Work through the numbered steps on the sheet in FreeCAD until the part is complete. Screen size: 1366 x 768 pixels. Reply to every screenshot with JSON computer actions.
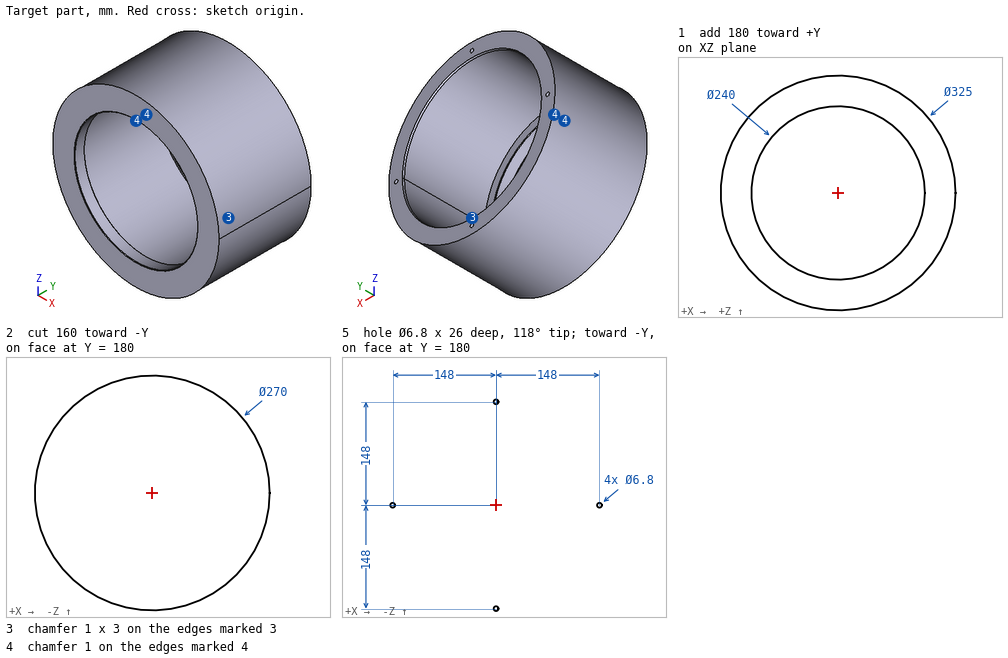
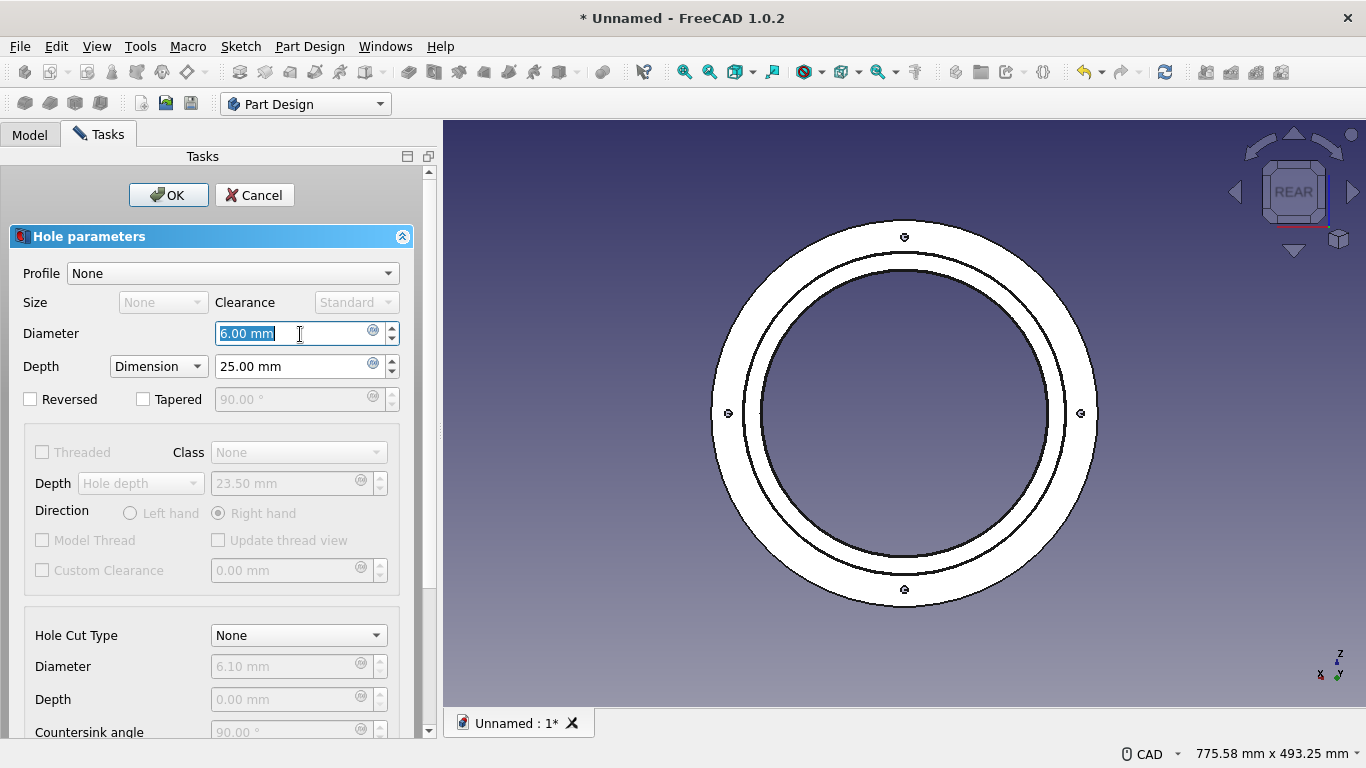
{"action": "type", "text": "6.8"}
{"action": "key", "text": "Tab"}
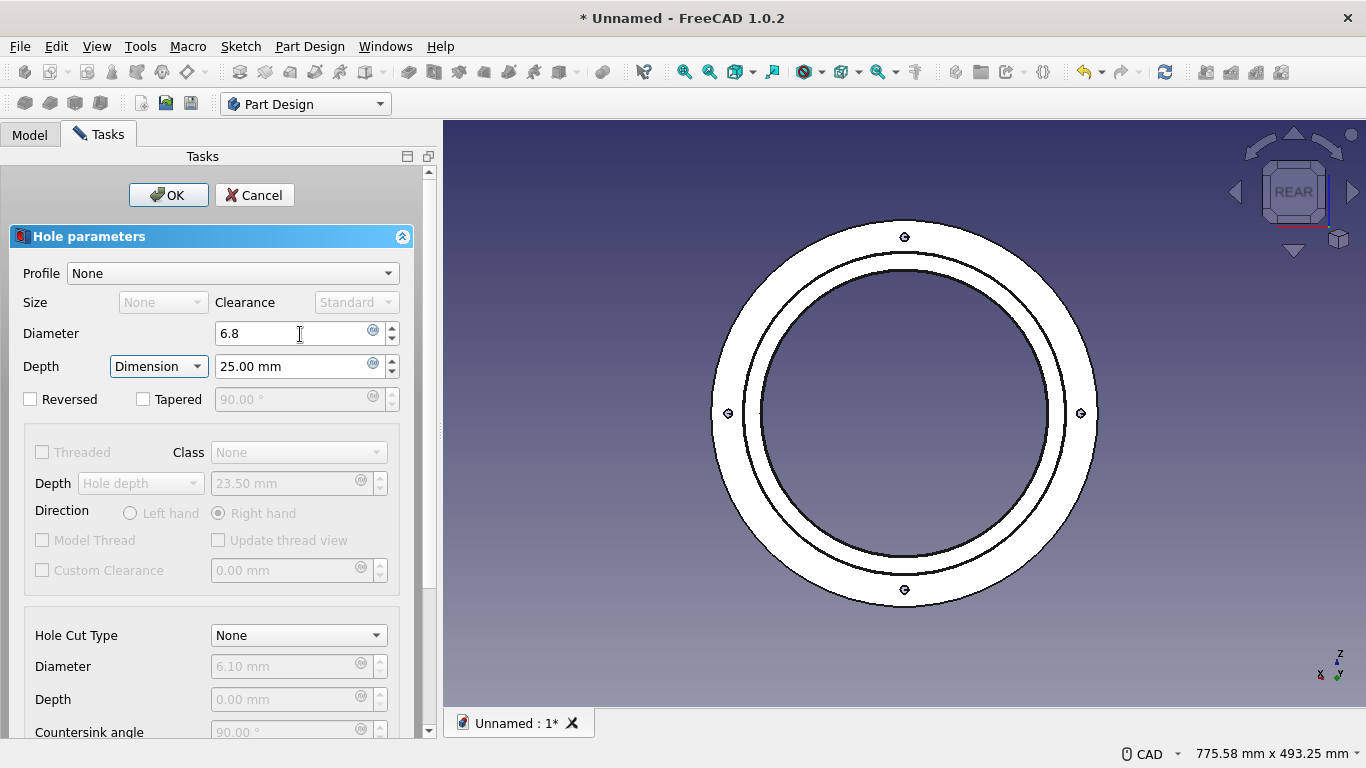
{"action": "triple_click", "coordinate": [300, 366]}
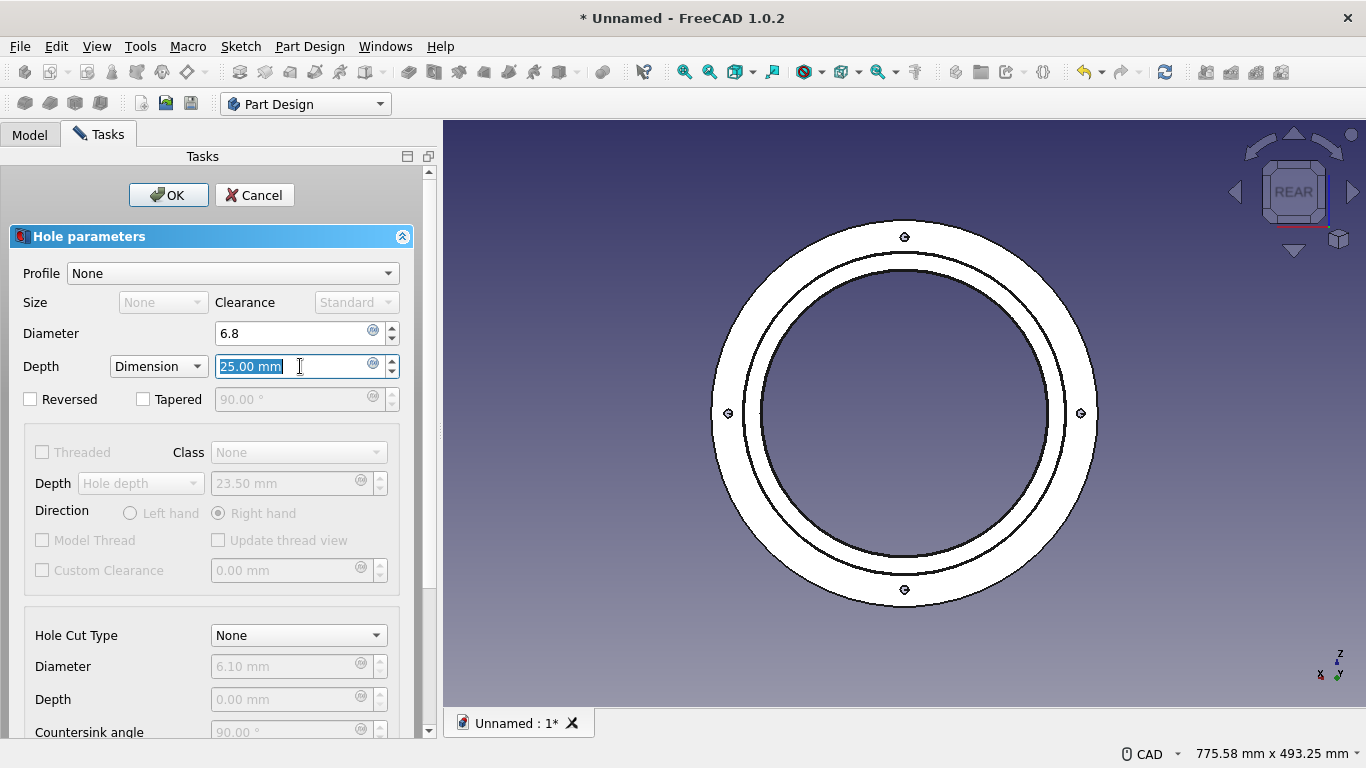
{"action": "type", "text": "26"}
{"action": "key", "text": "Tab"}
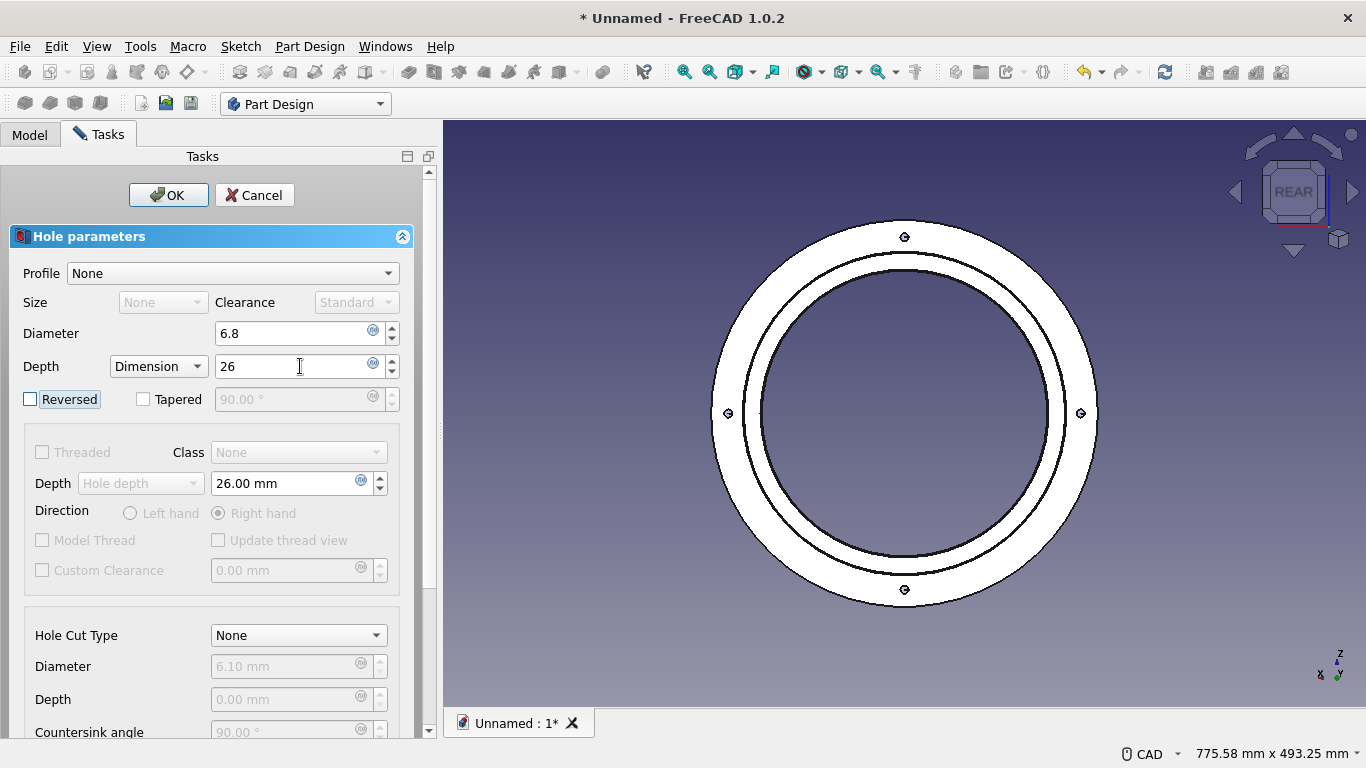
{"action": "left_click", "coordinate": [169, 195]}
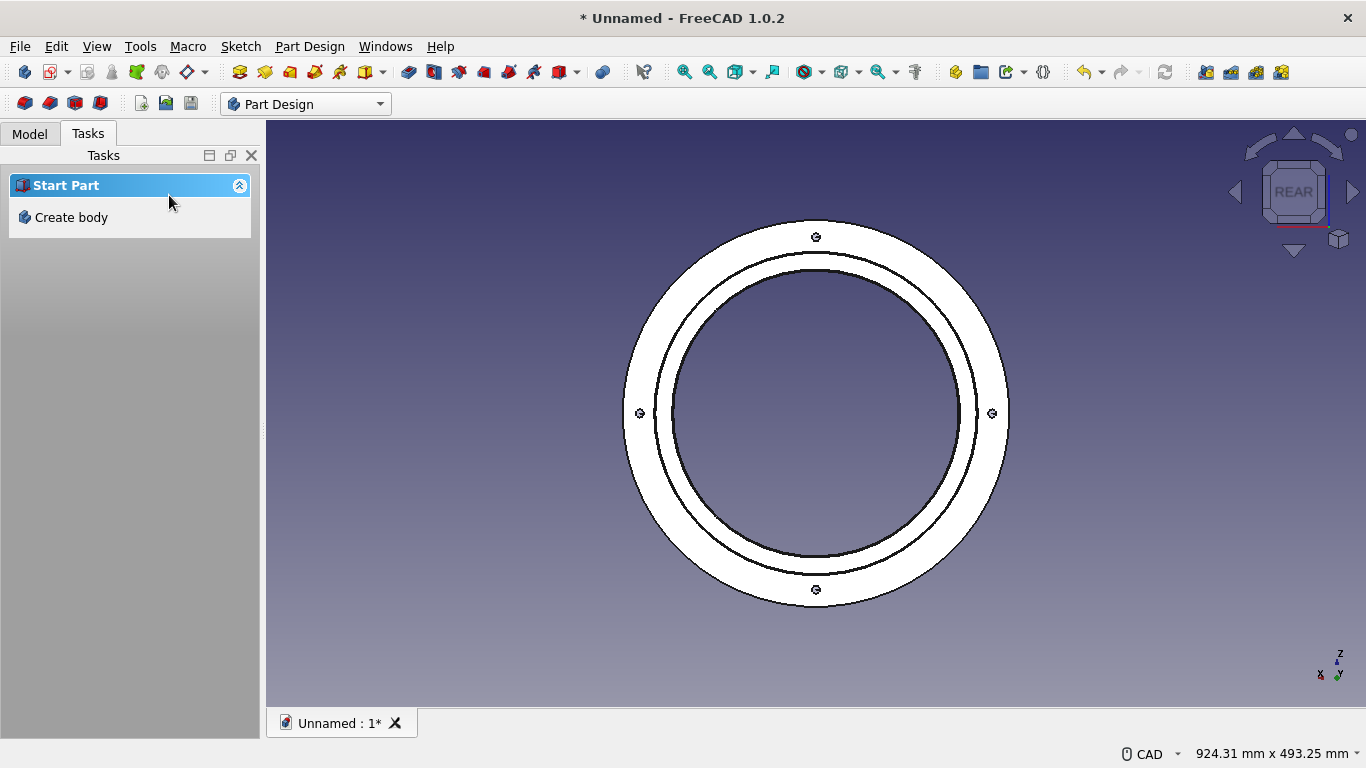
{"action": "key", "text": "0"}